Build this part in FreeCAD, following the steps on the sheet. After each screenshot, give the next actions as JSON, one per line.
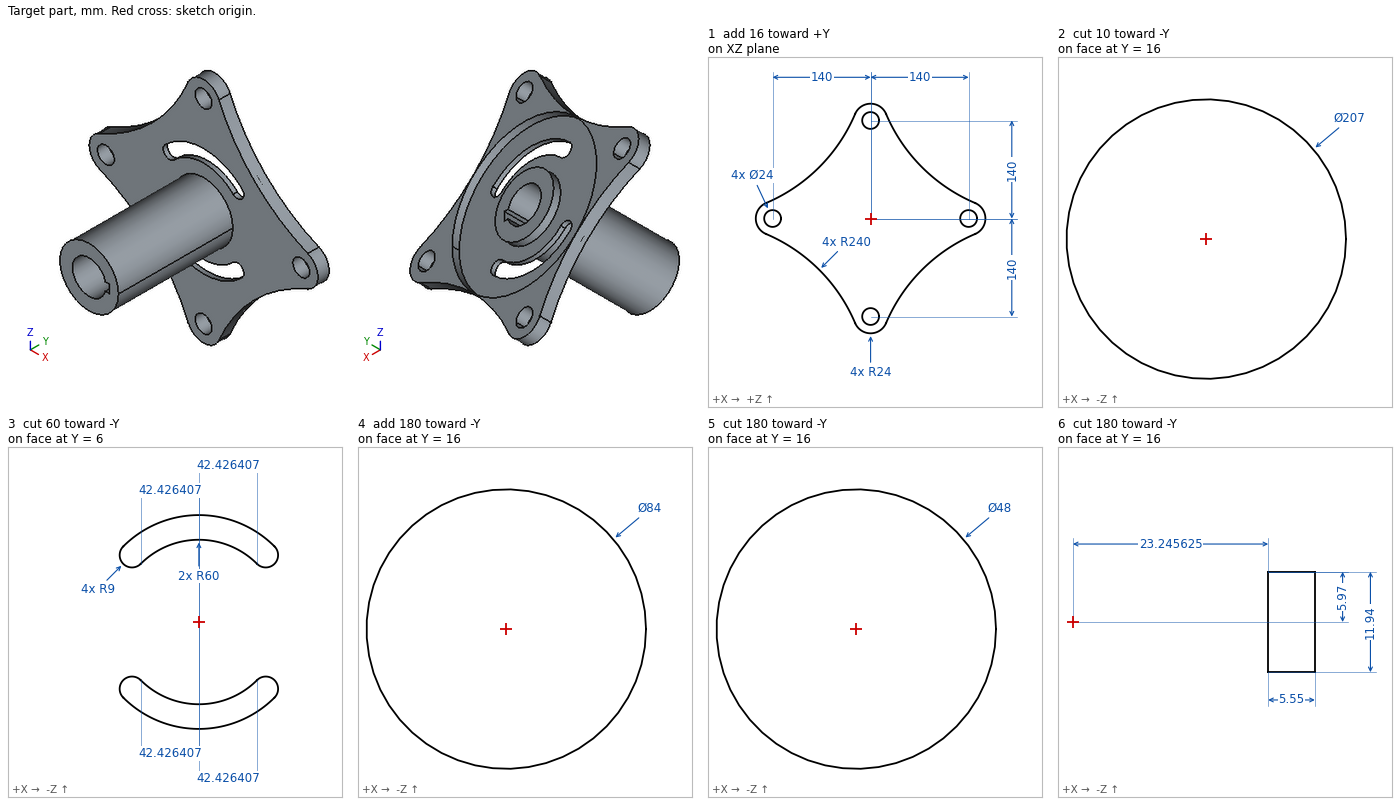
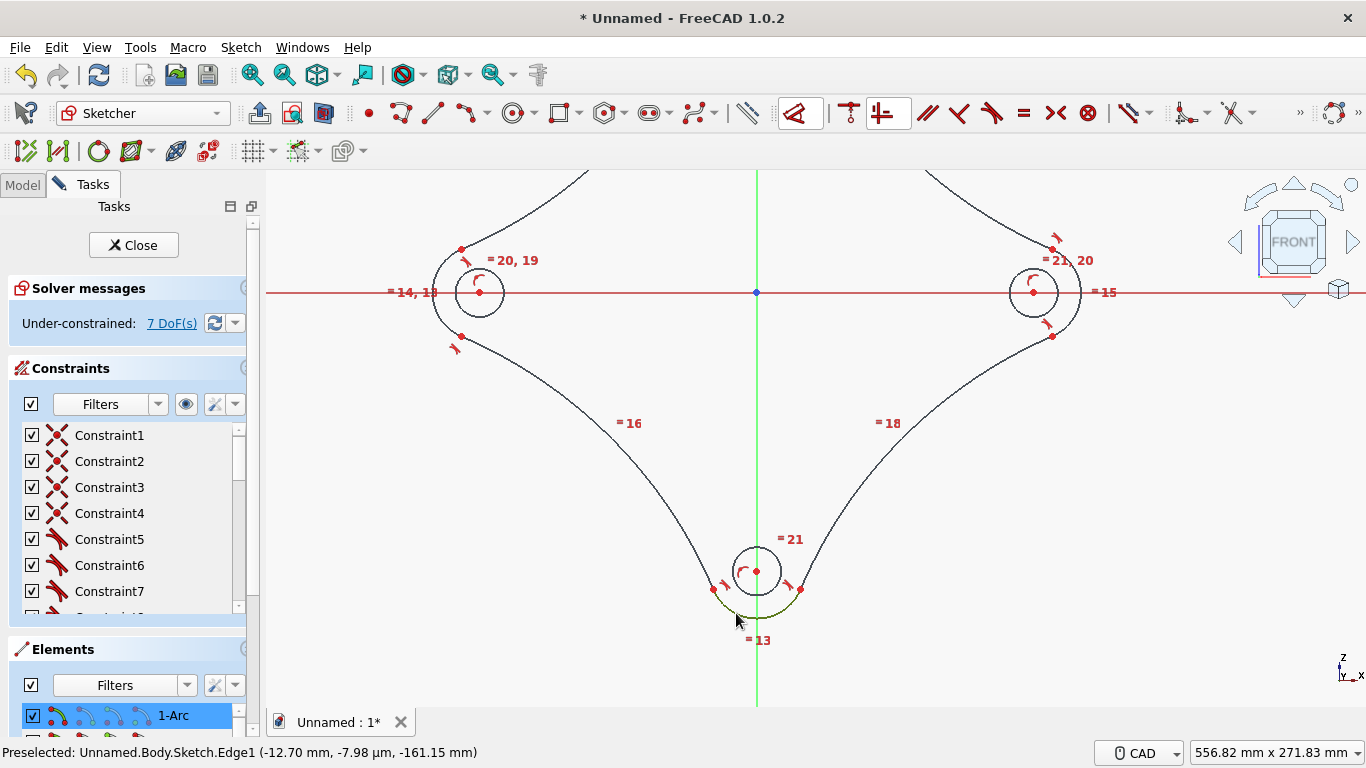
{"action": "left_click", "coordinate": [818, 114]}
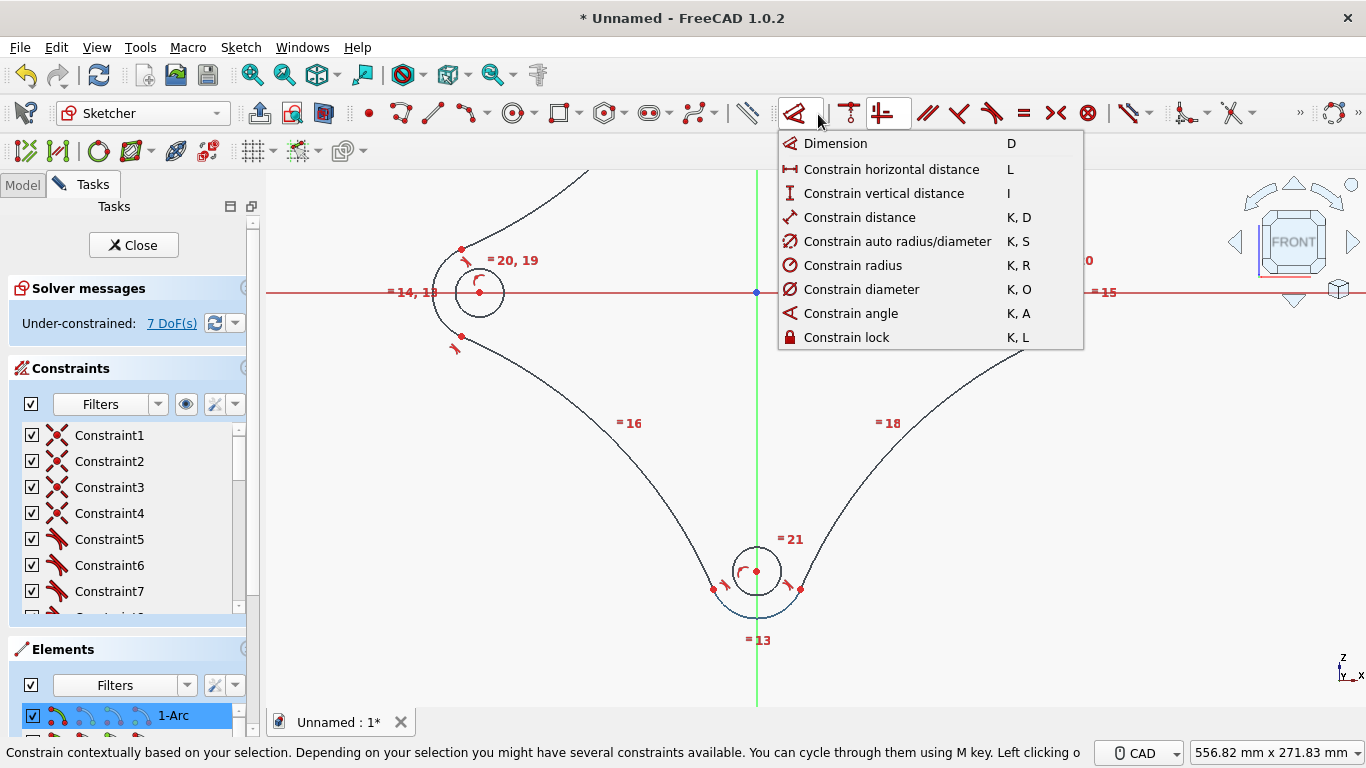
{"action": "left_click", "coordinate": [931, 265]}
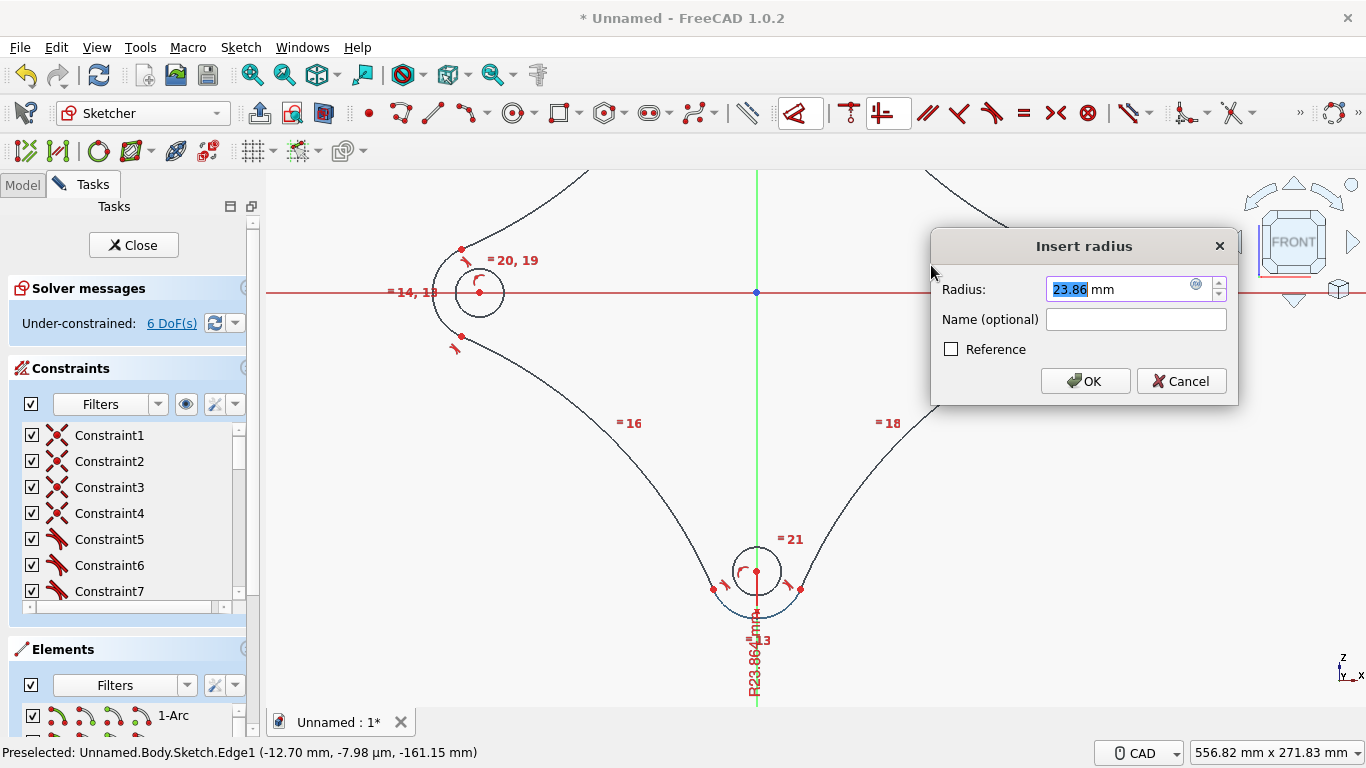
{"action": "type", "text": "24"}
{"action": "key", "text": "Return"}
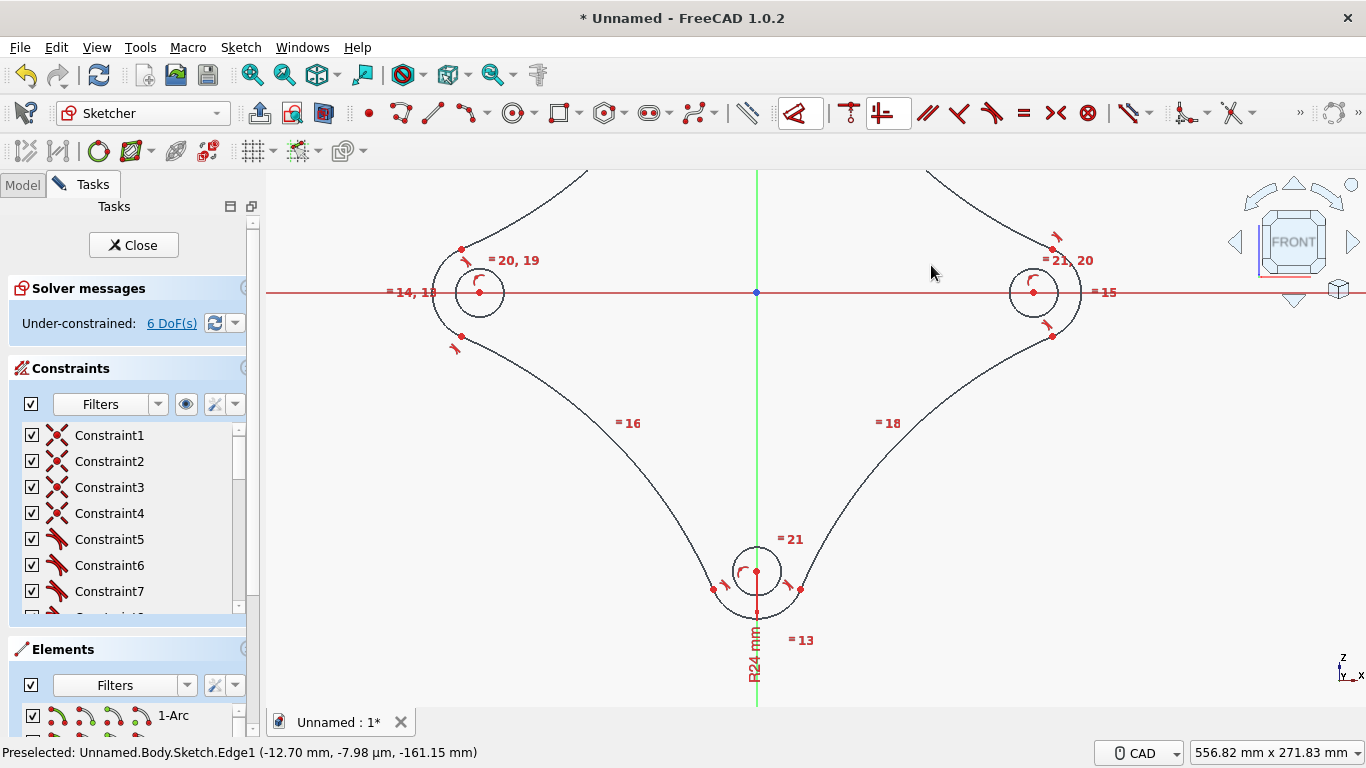
{"action": "left_click", "coordinate": [659, 495]}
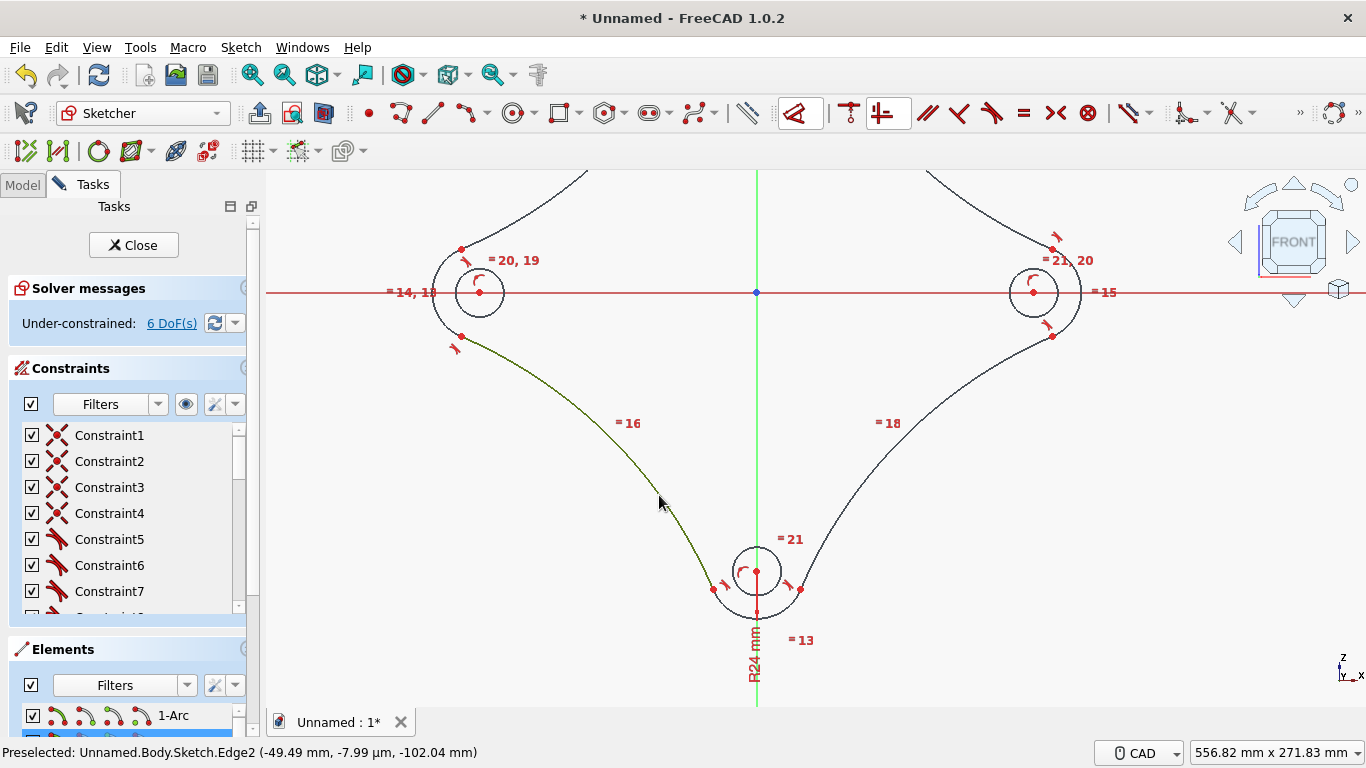
{"action": "left_click", "coordinate": [818, 114]}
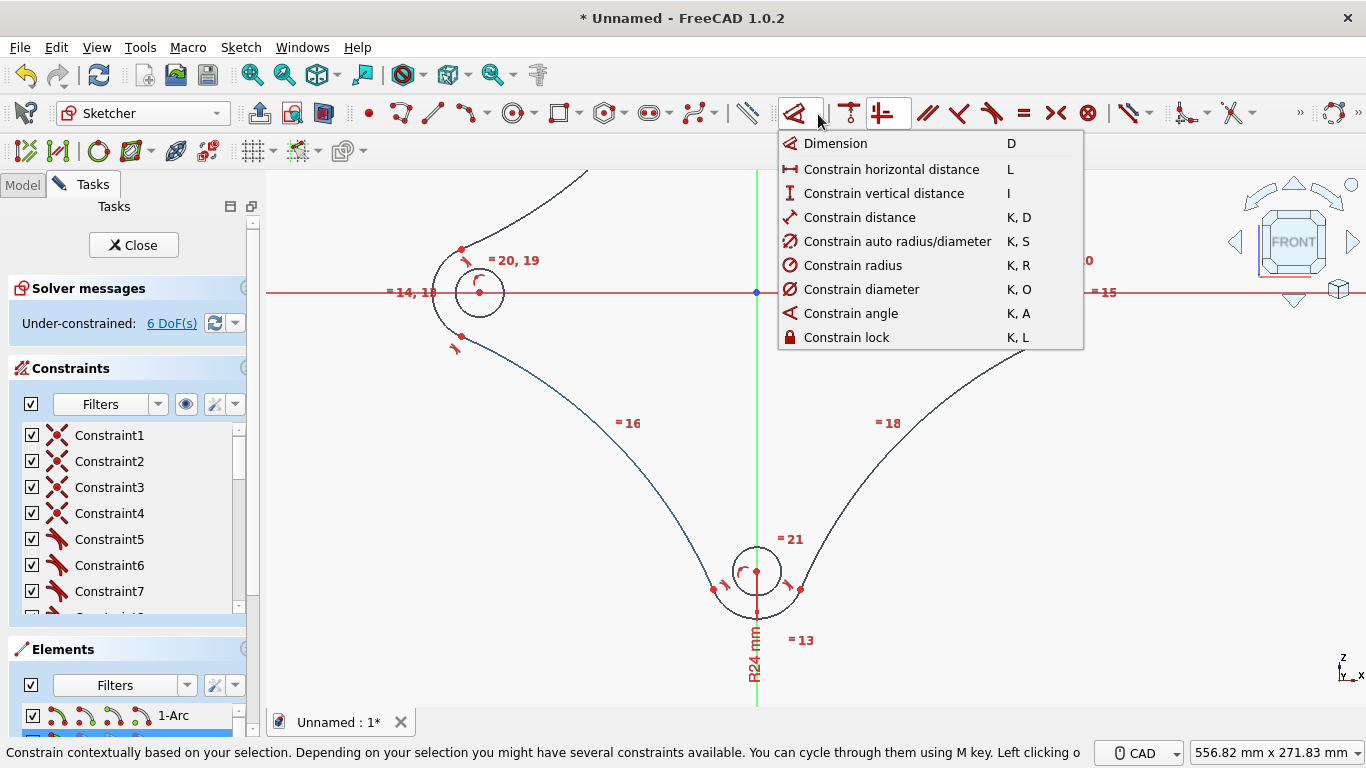
{"action": "left_click", "coordinate": [931, 265]}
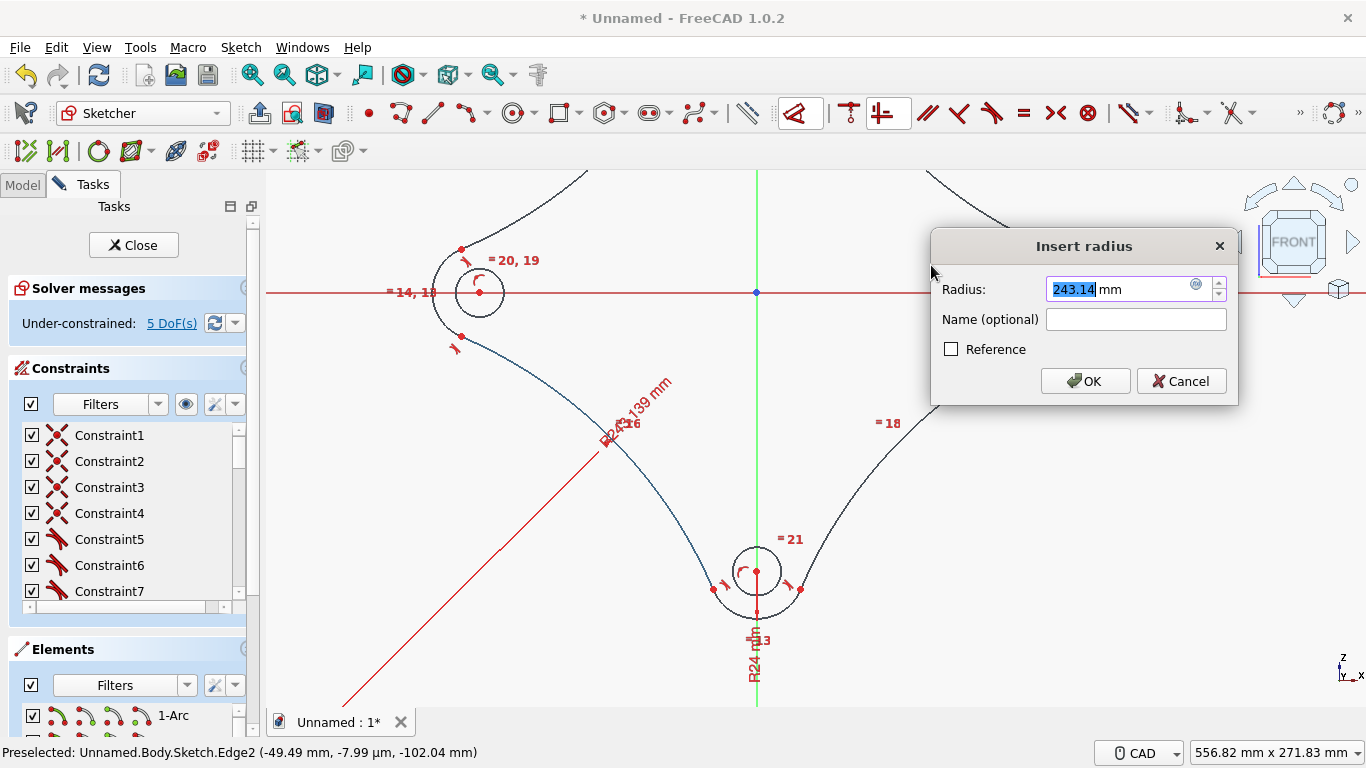
{"action": "type", "text": "240"}
{"action": "key", "text": "Return"}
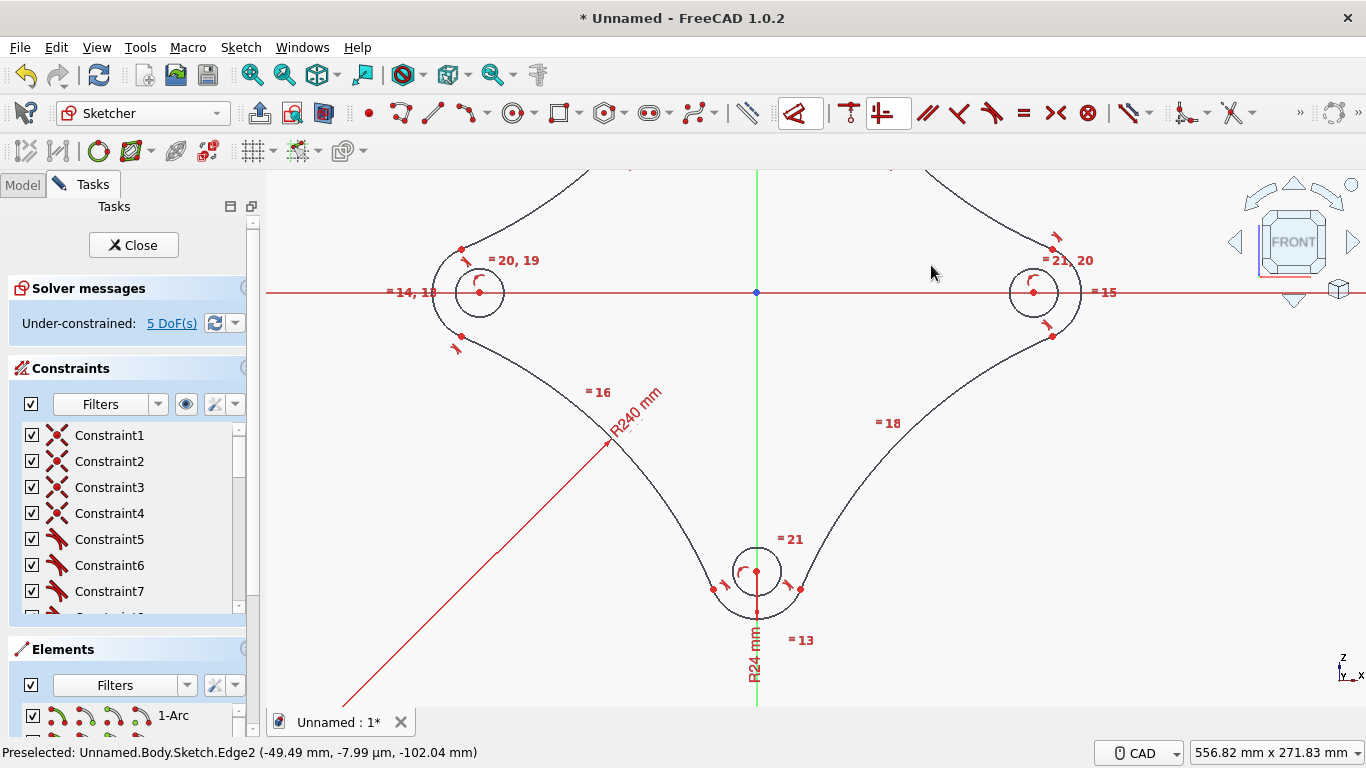
{"action": "scroll", "coordinate": [736, 616], "scroll_direction": "down", "scroll_amount": 3}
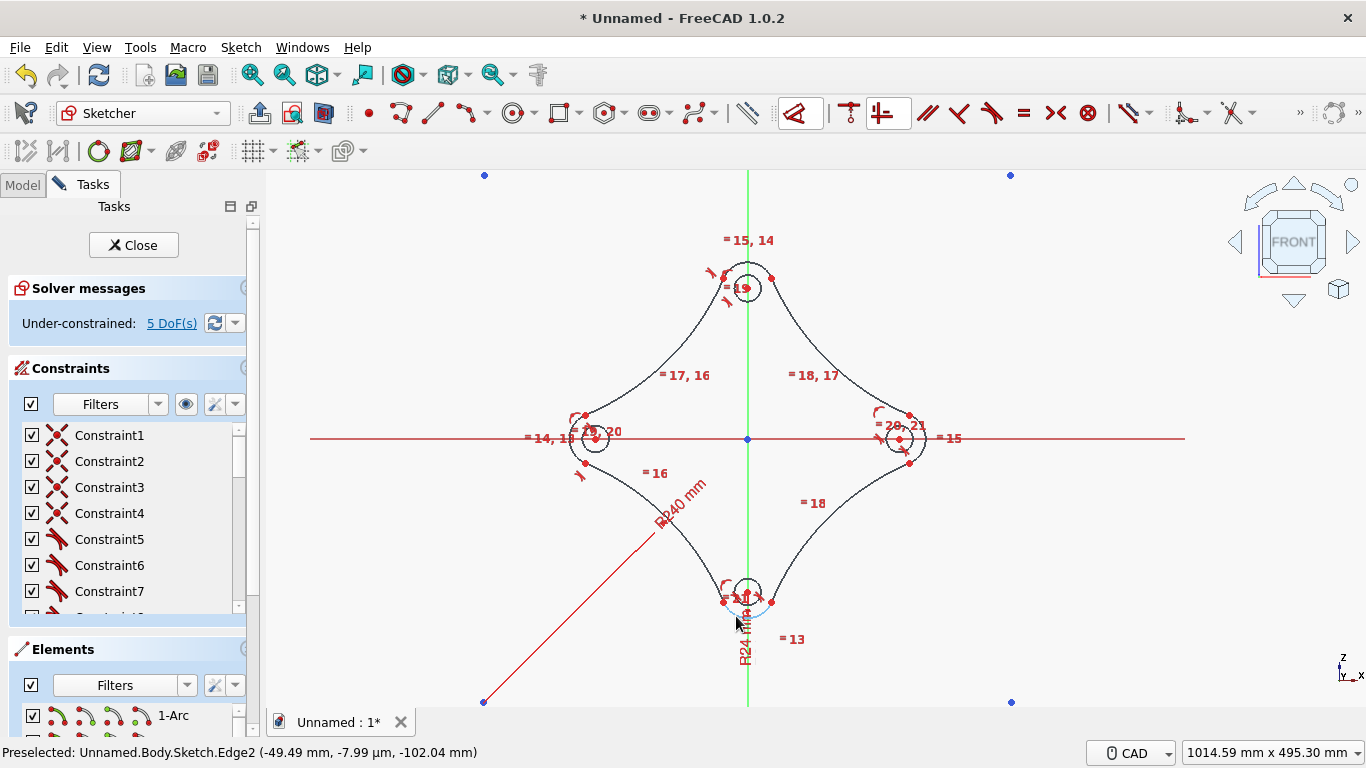
{"action": "scroll", "coordinate": [757, 279], "scroll_direction": "up", "scroll_amount": 3}